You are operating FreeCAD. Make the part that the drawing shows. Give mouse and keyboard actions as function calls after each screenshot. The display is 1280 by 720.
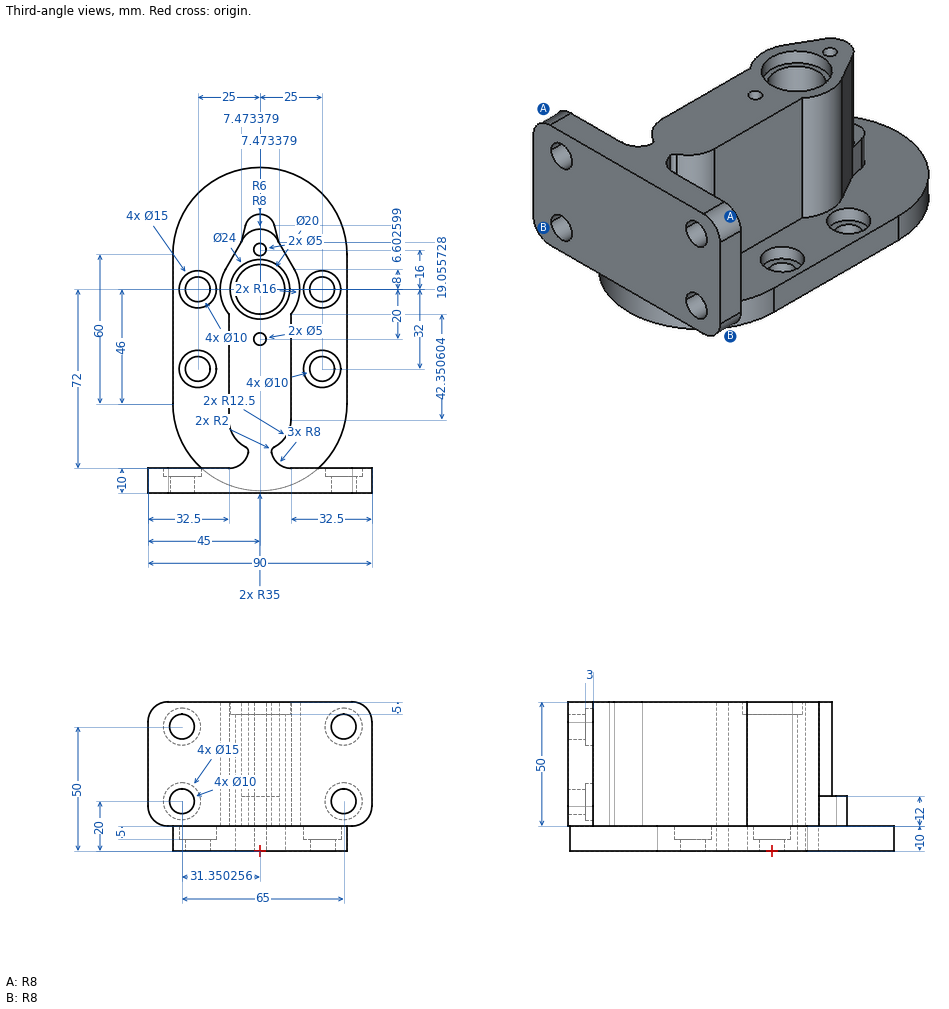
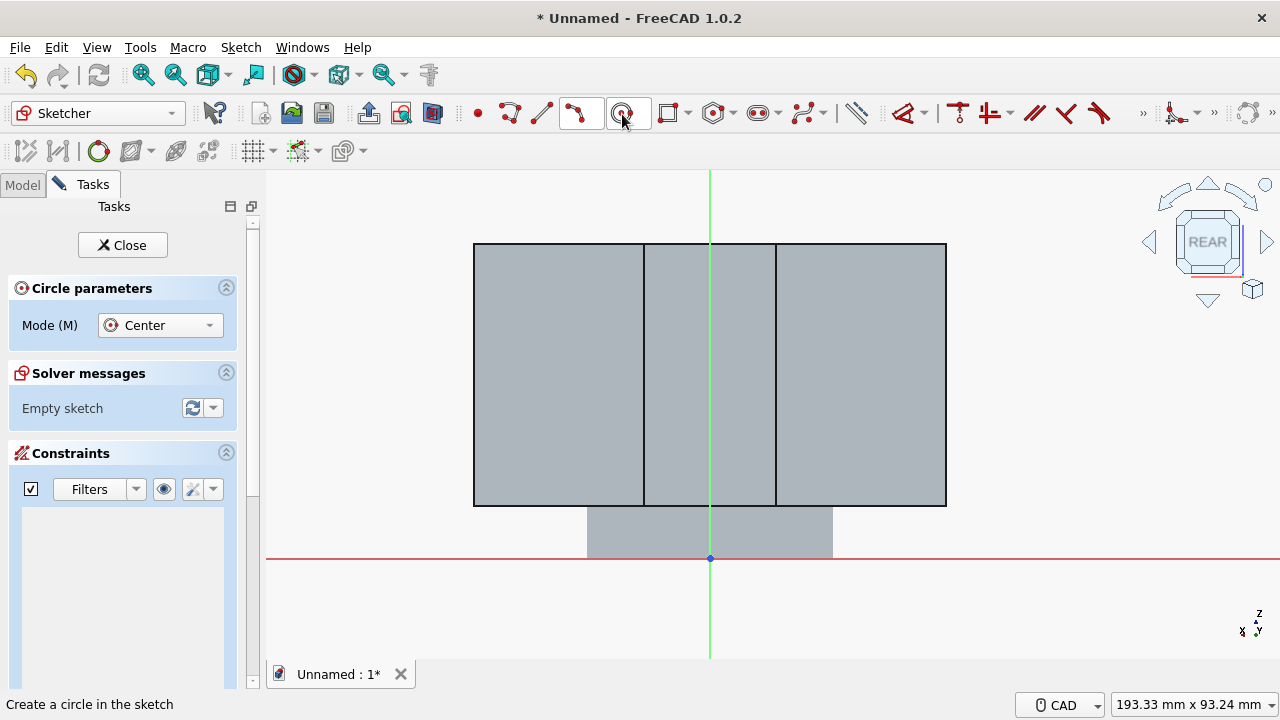
click(874, 454)
click(893, 435)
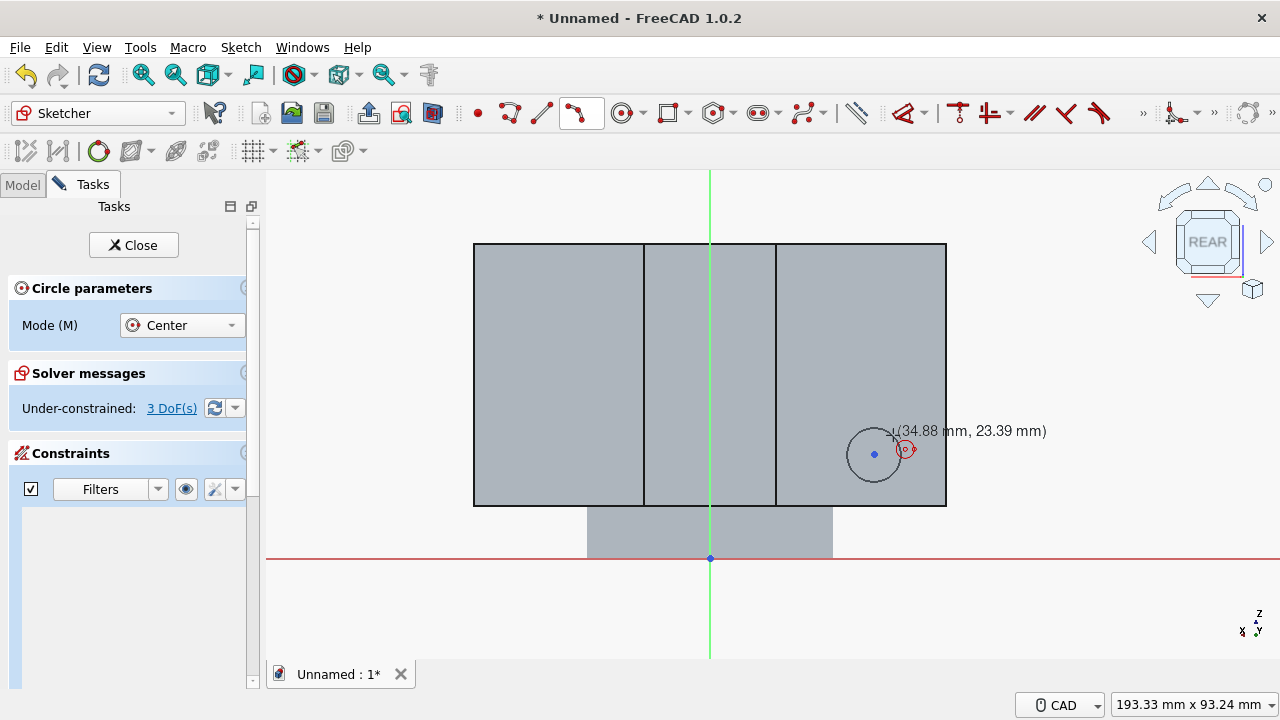
click(874, 296)
click(893, 278)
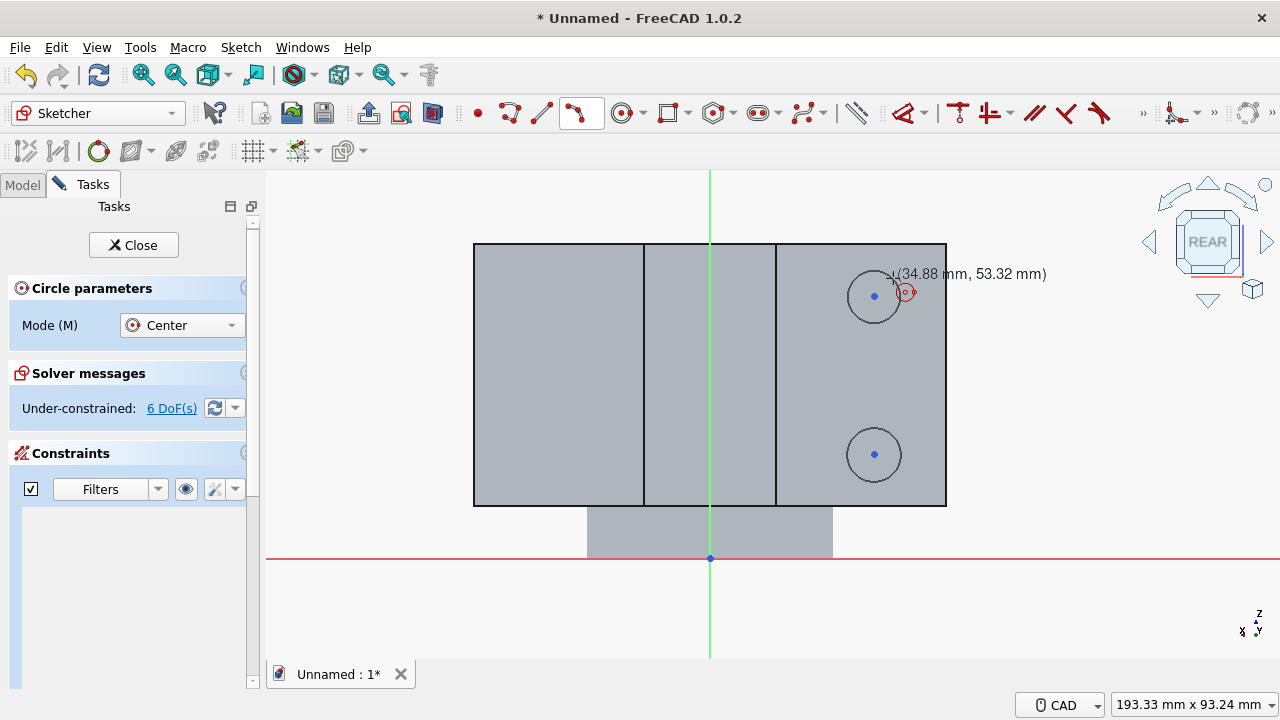
click(534, 454)
click(552, 435)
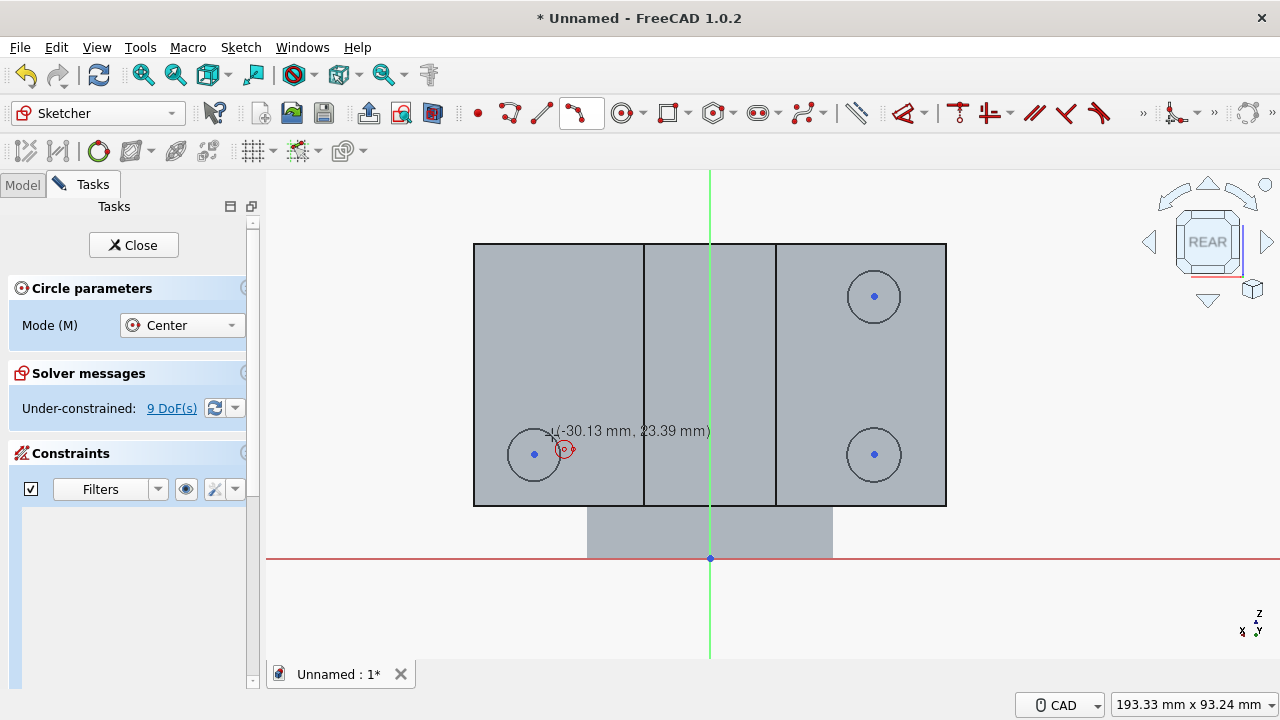
click(534, 296)
click(552, 278)
key(Escape)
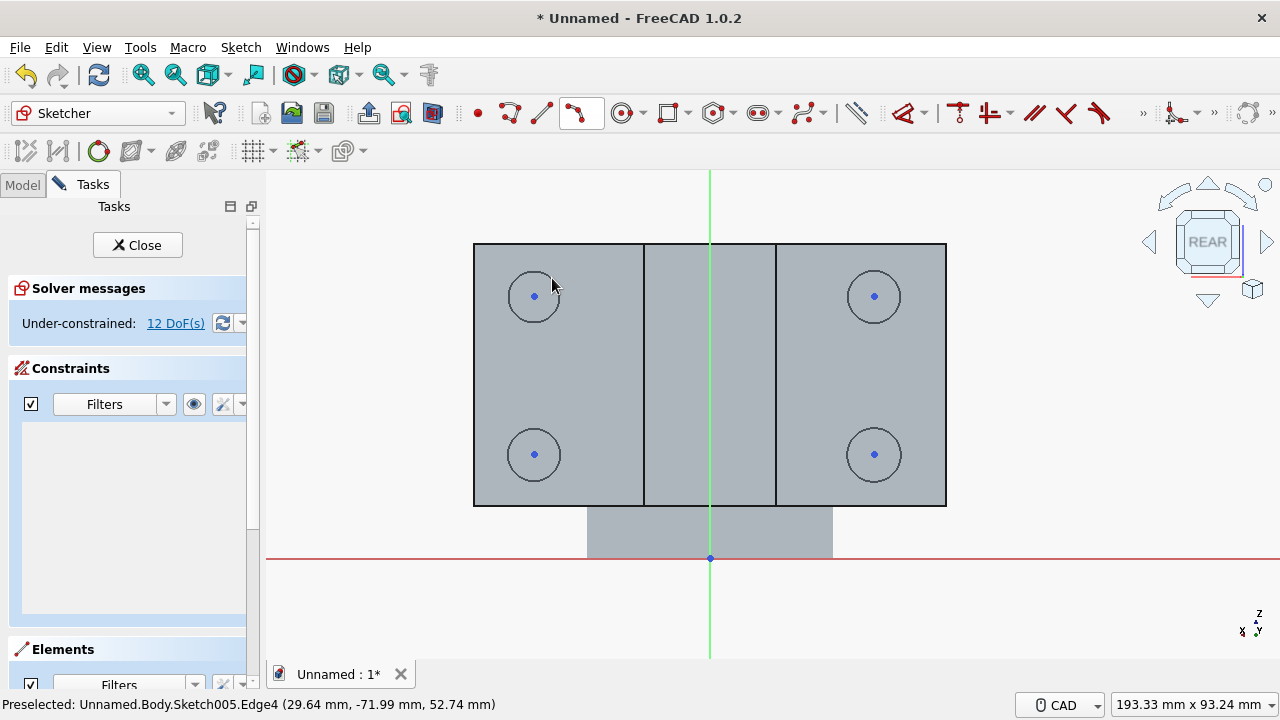
click(893, 436)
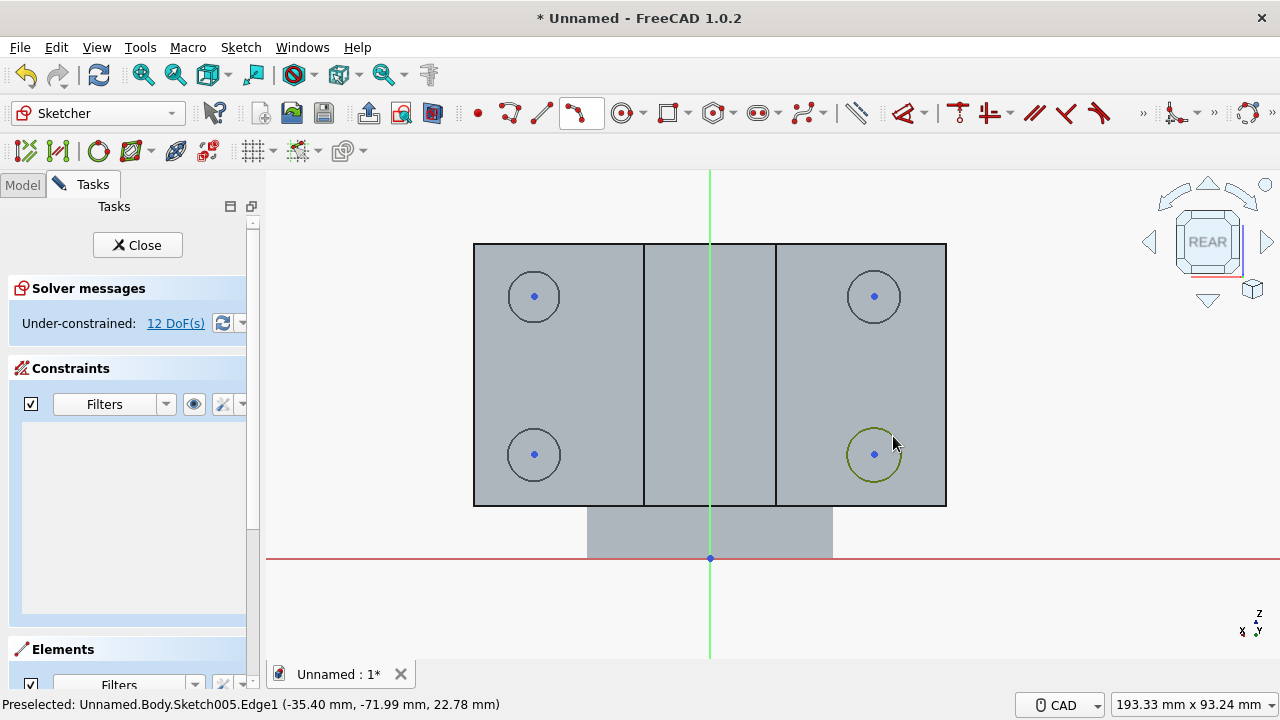
click(892, 278)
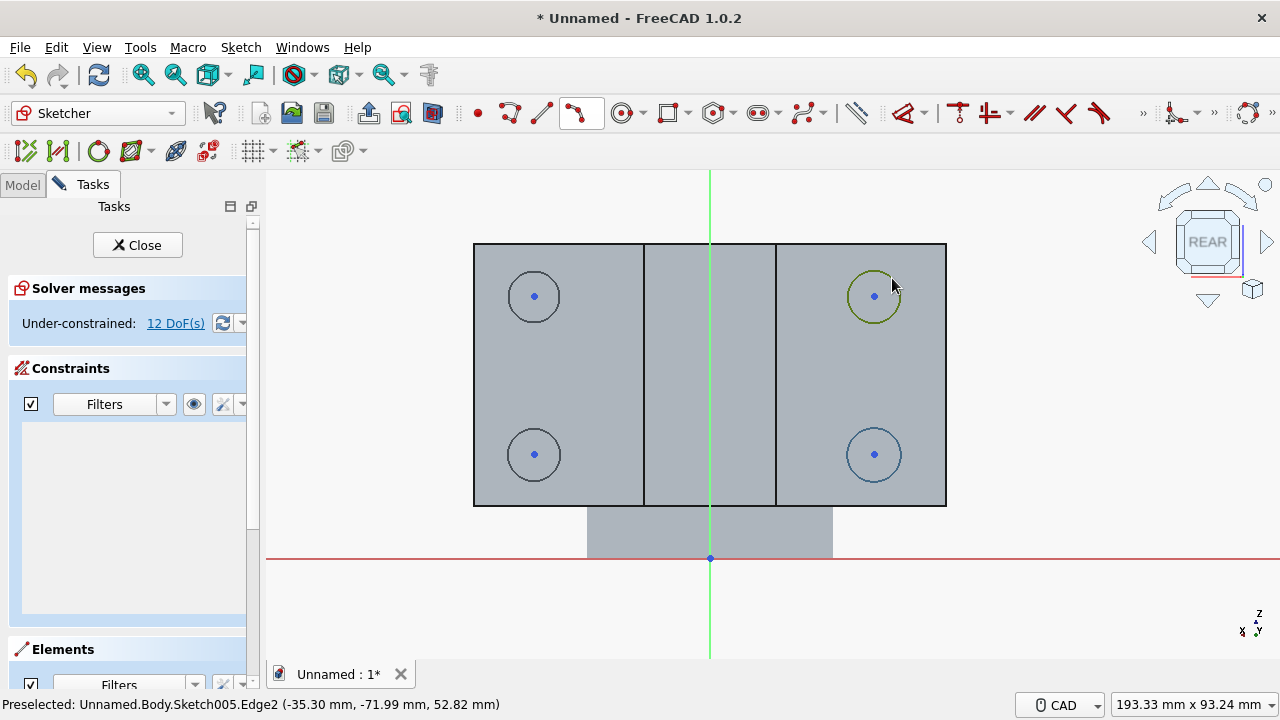
click(552, 436)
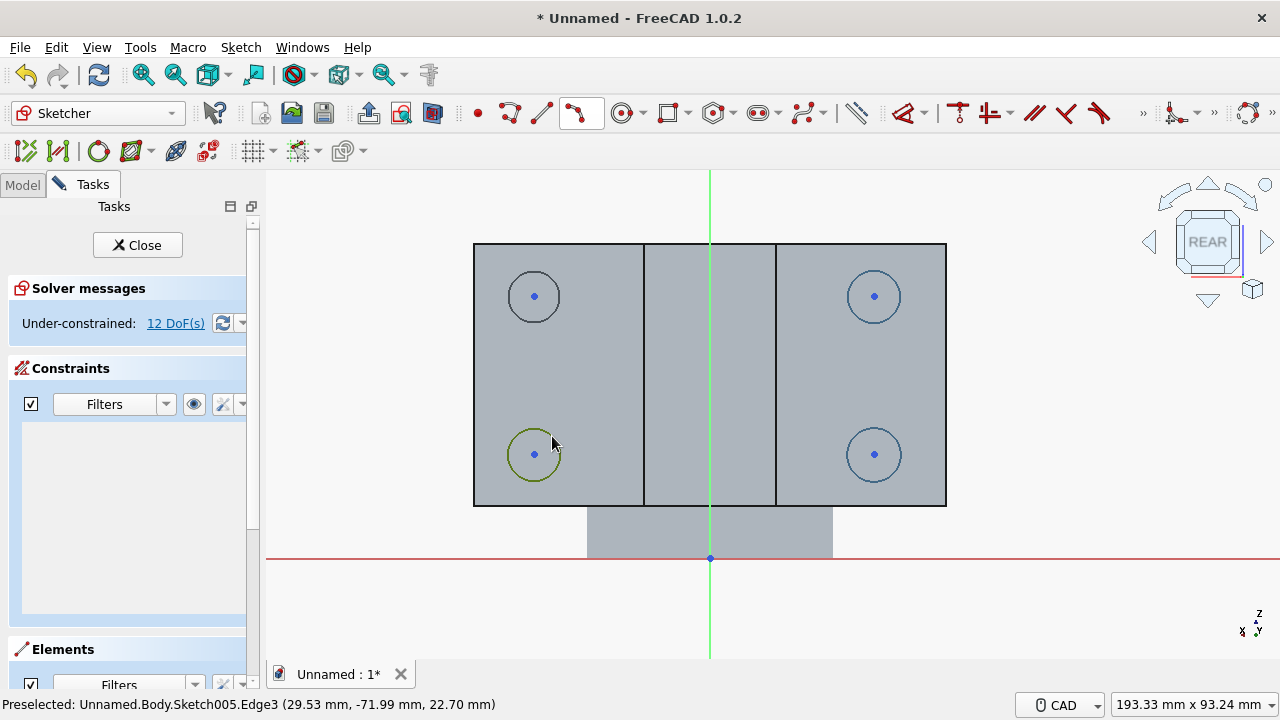
click(552, 279)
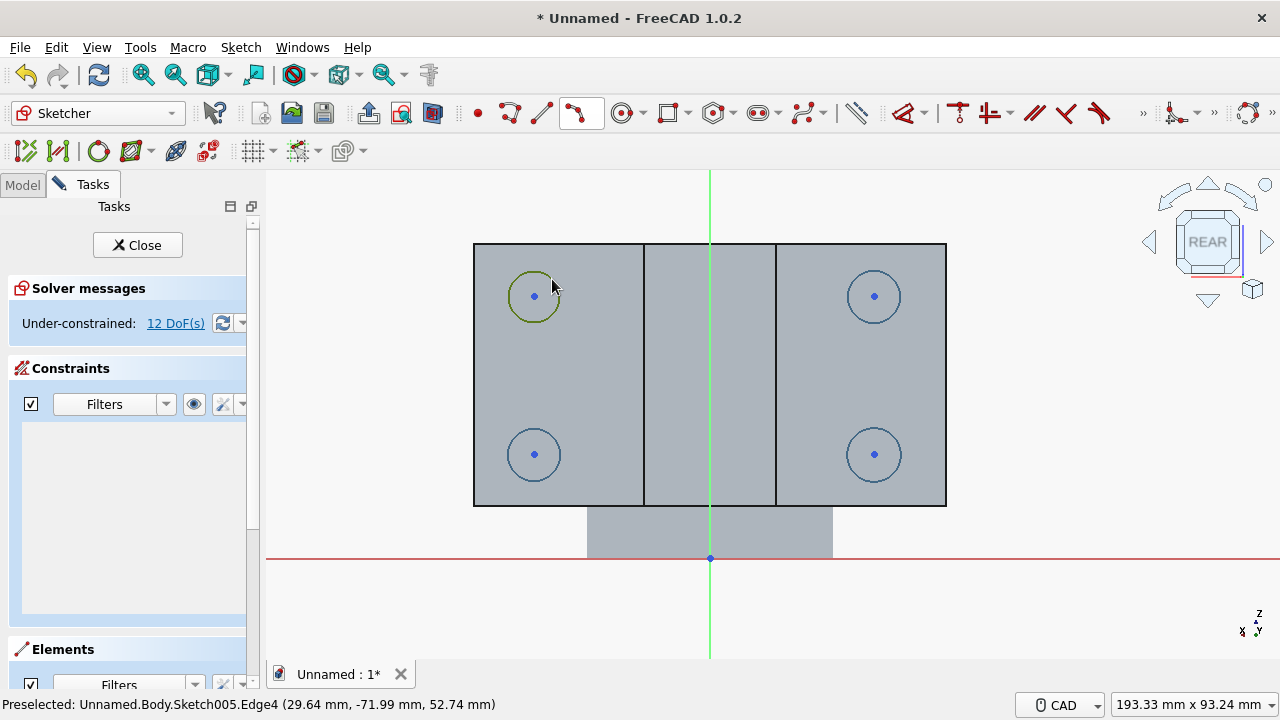
key(e)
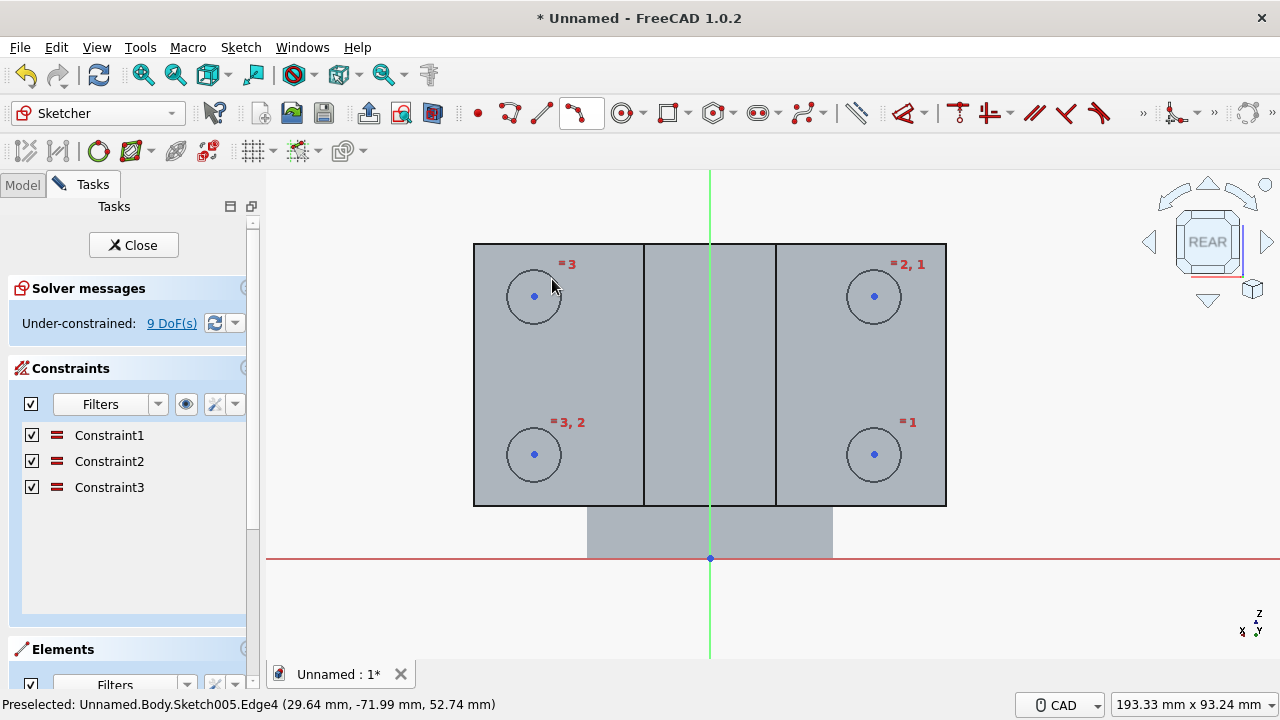
click(904, 114)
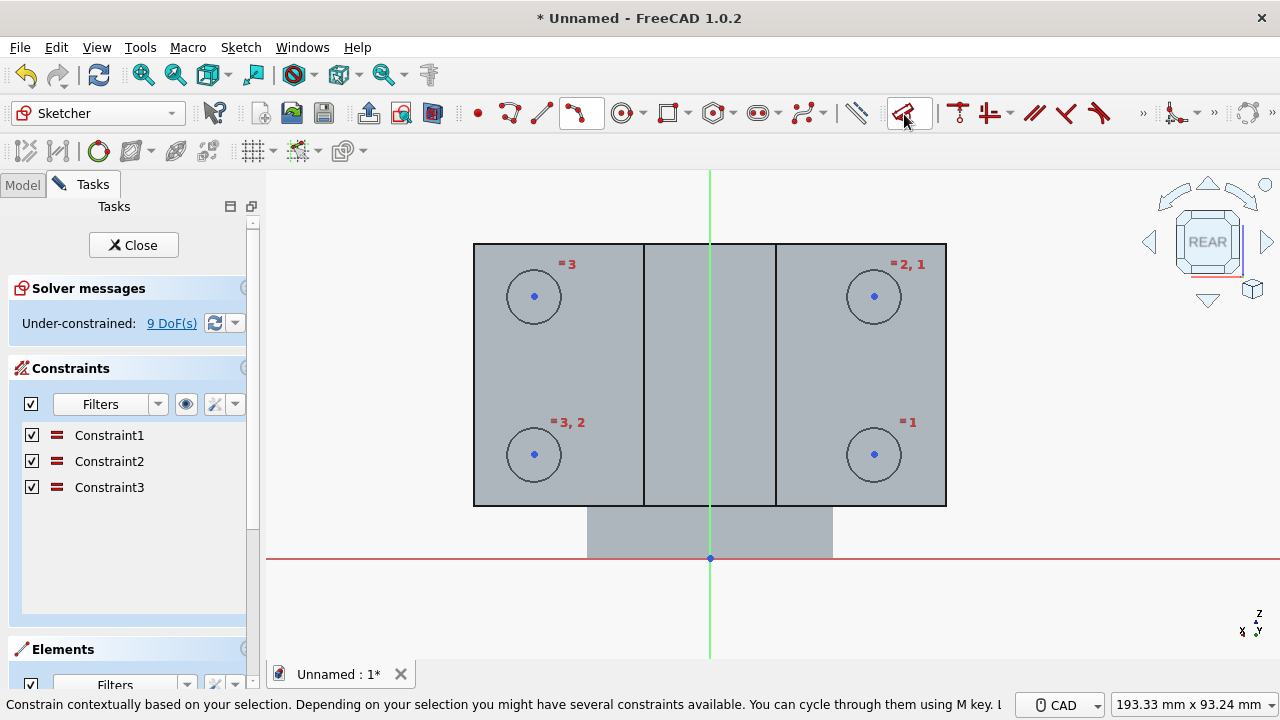
click(893, 436)
click(916, 413)